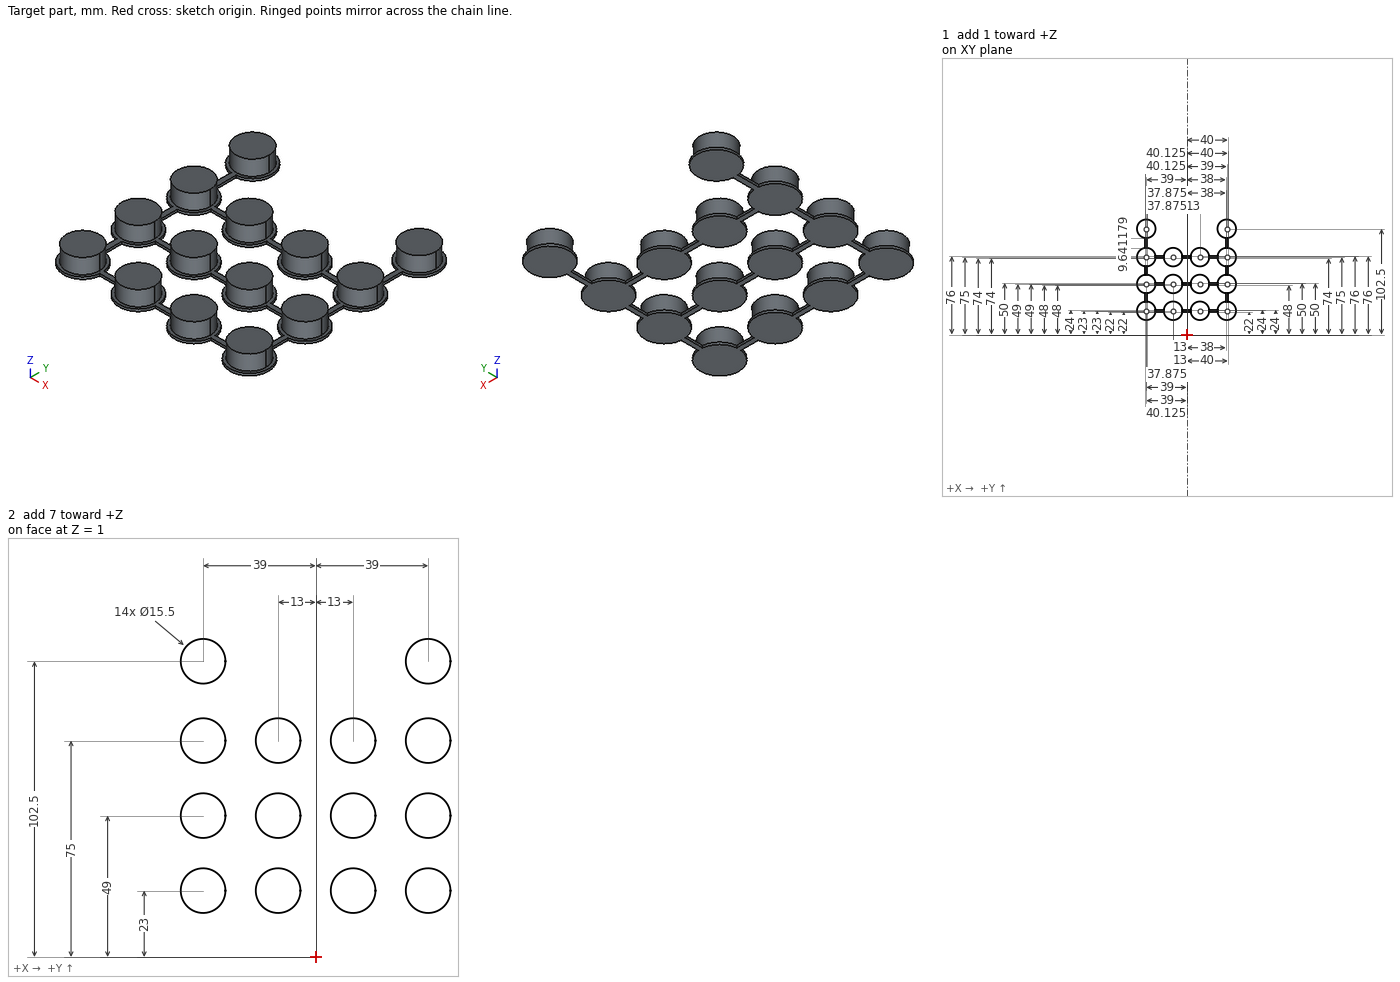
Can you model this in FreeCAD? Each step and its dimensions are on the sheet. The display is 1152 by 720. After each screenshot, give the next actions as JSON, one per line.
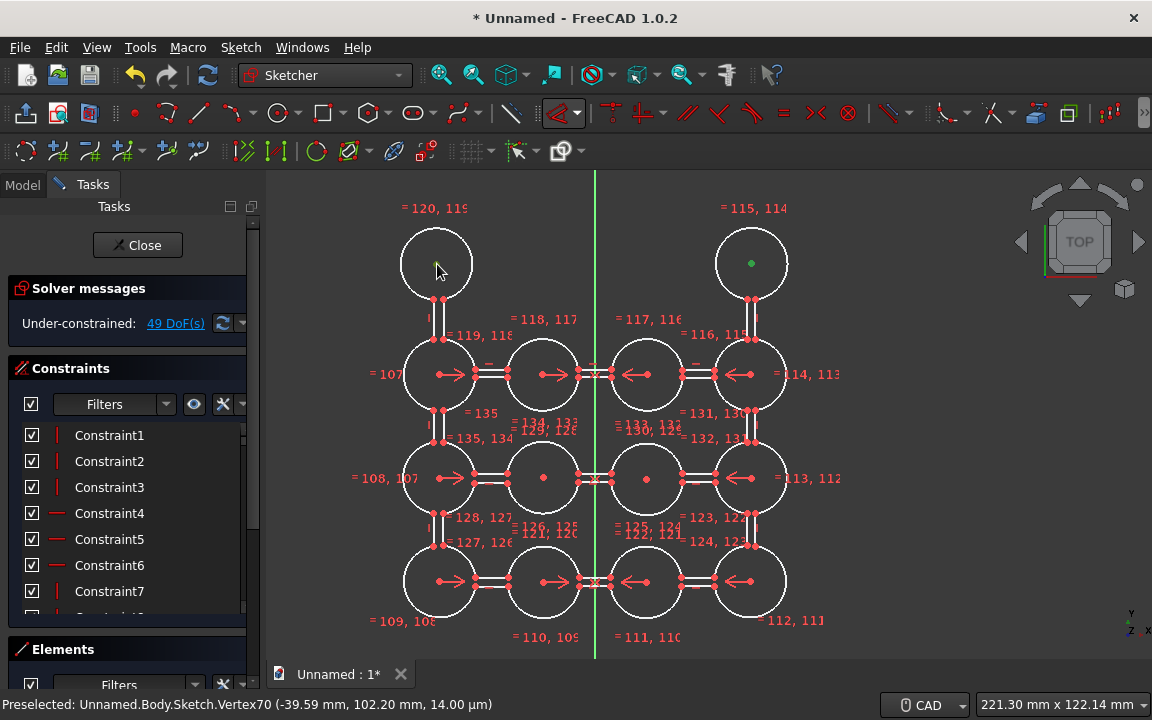
{"action": "left_click", "coordinate": [595, 538]}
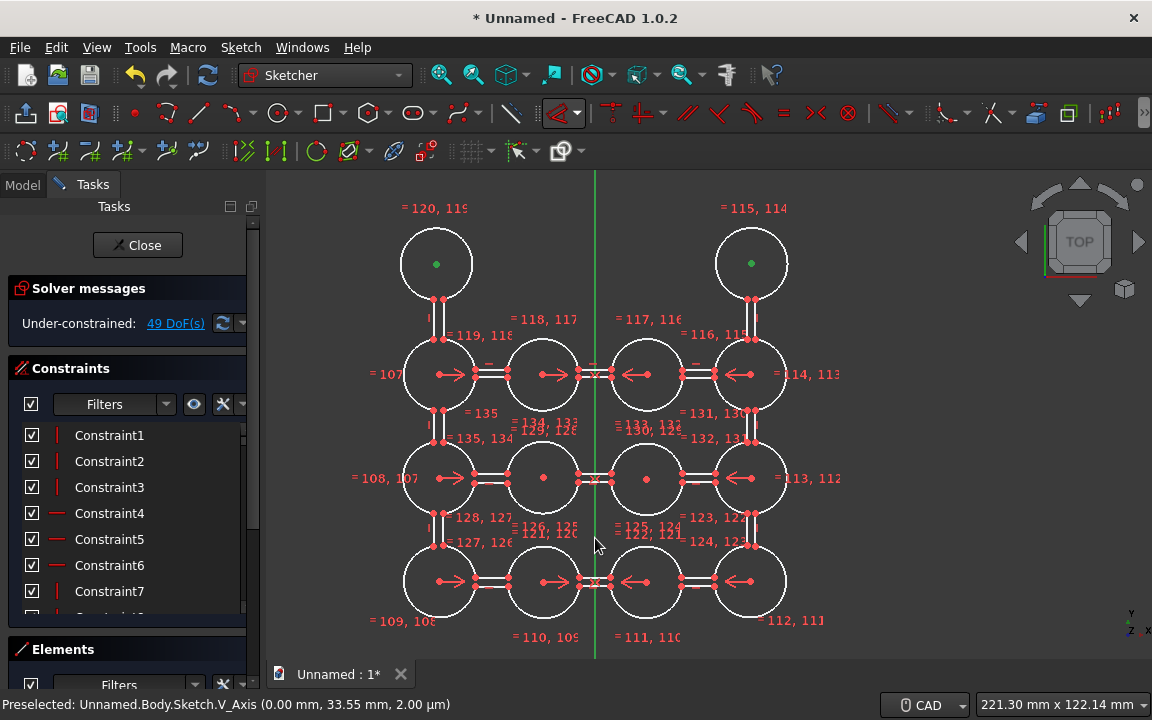
{"action": "left_click", "coordinate": [816, 114]}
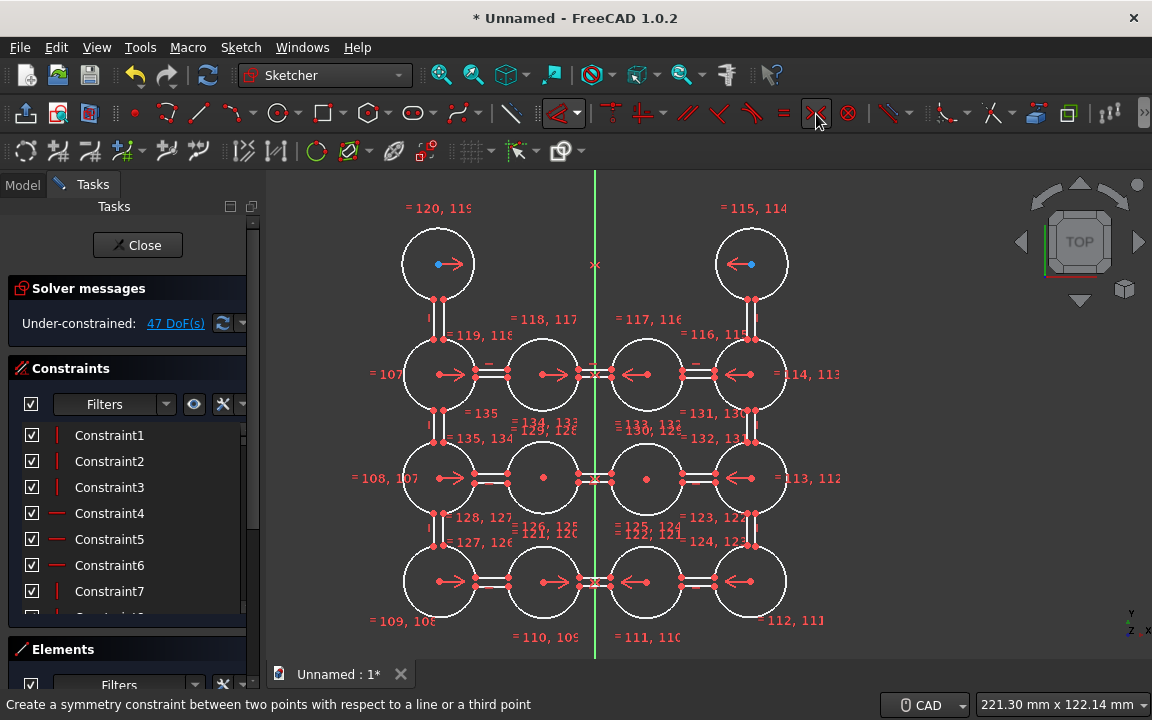
{"action": "left_click", "coordinate": [543, 478]}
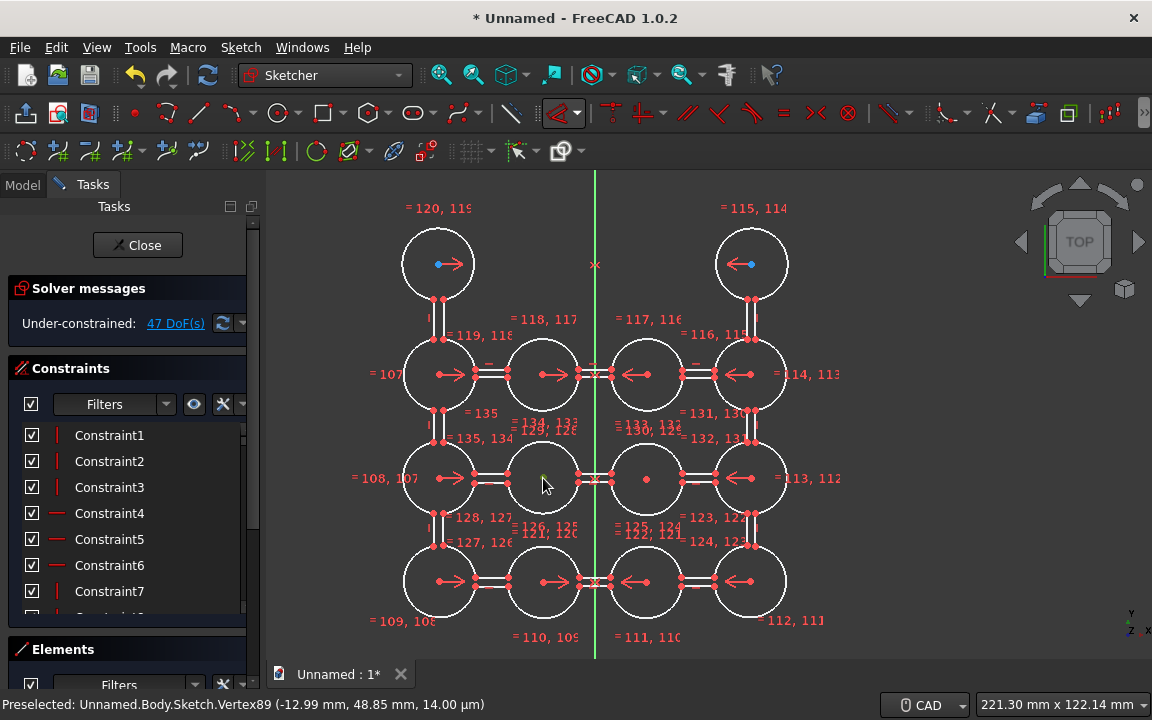
{"action": "left_click", "coordinate": [647, 479]}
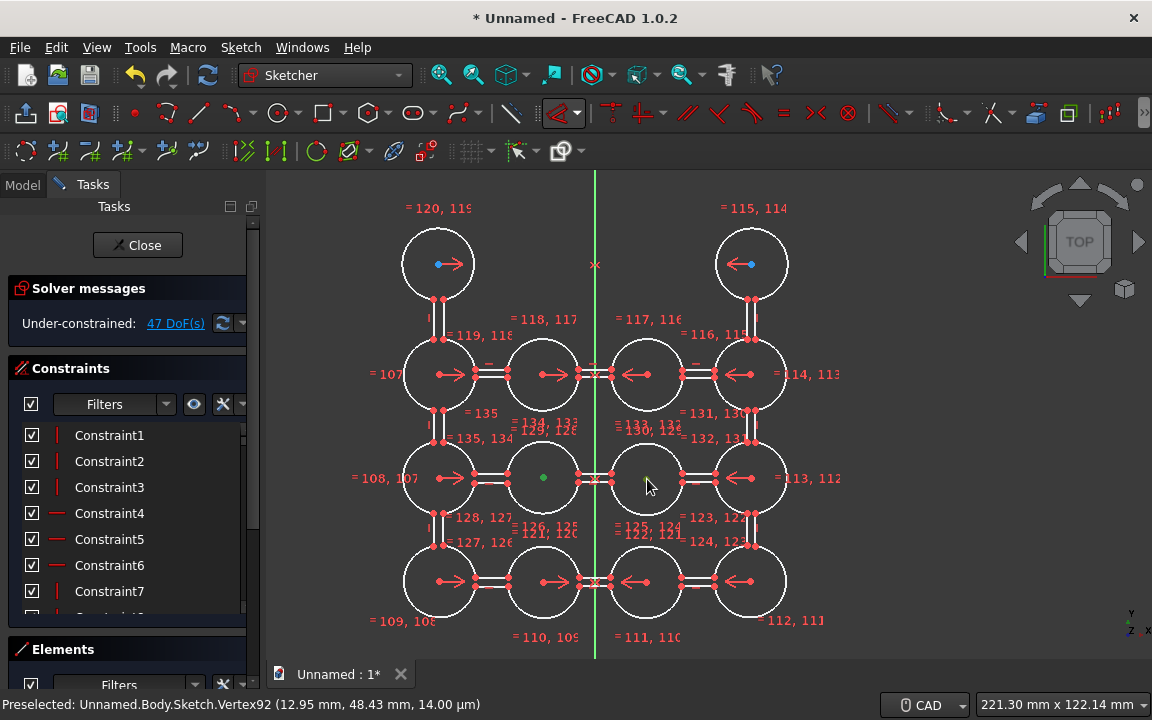
{"action": "left_click", "coordinate": [595, 538]}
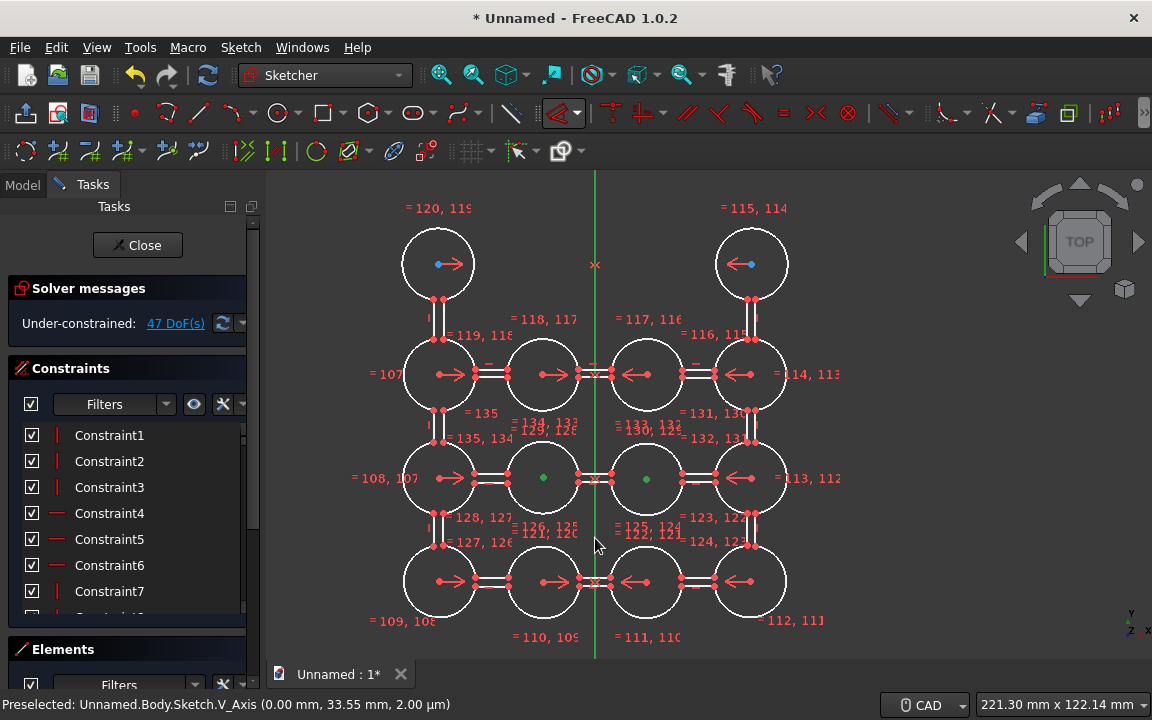
{"action": "left_click", "coordinate": [816, 114]}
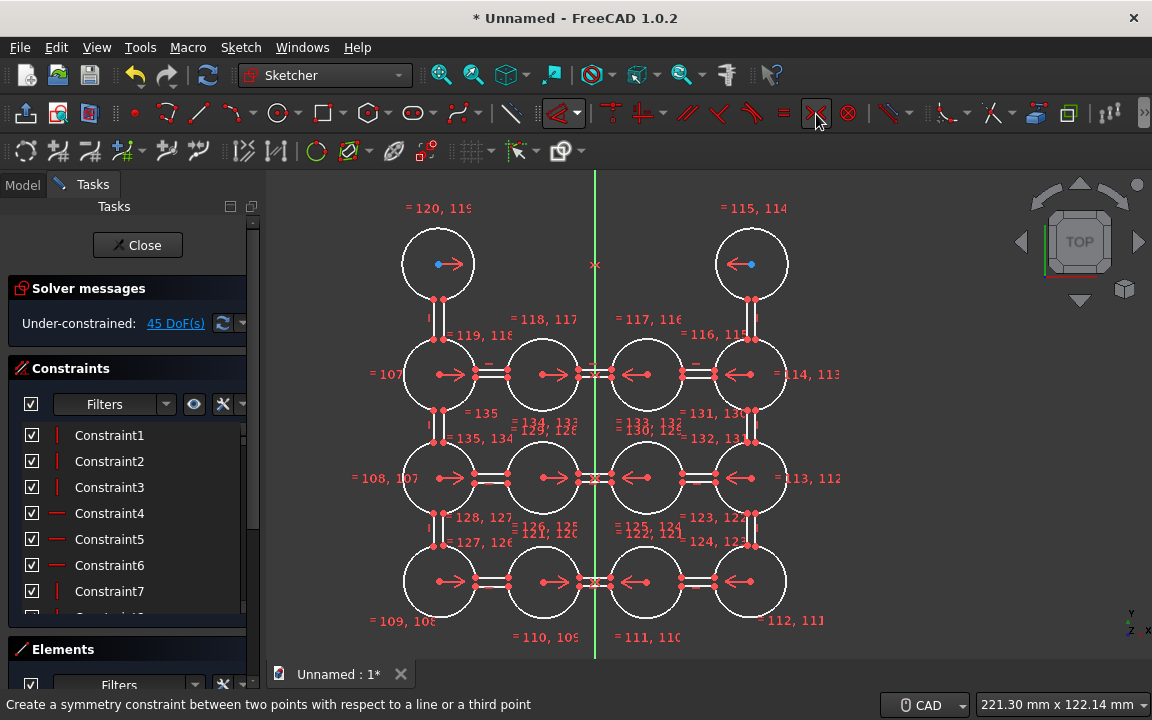
{"action": "scroll", "coordinate": [475, 587], "scroll_direction": "up", "scroll_amount": 2}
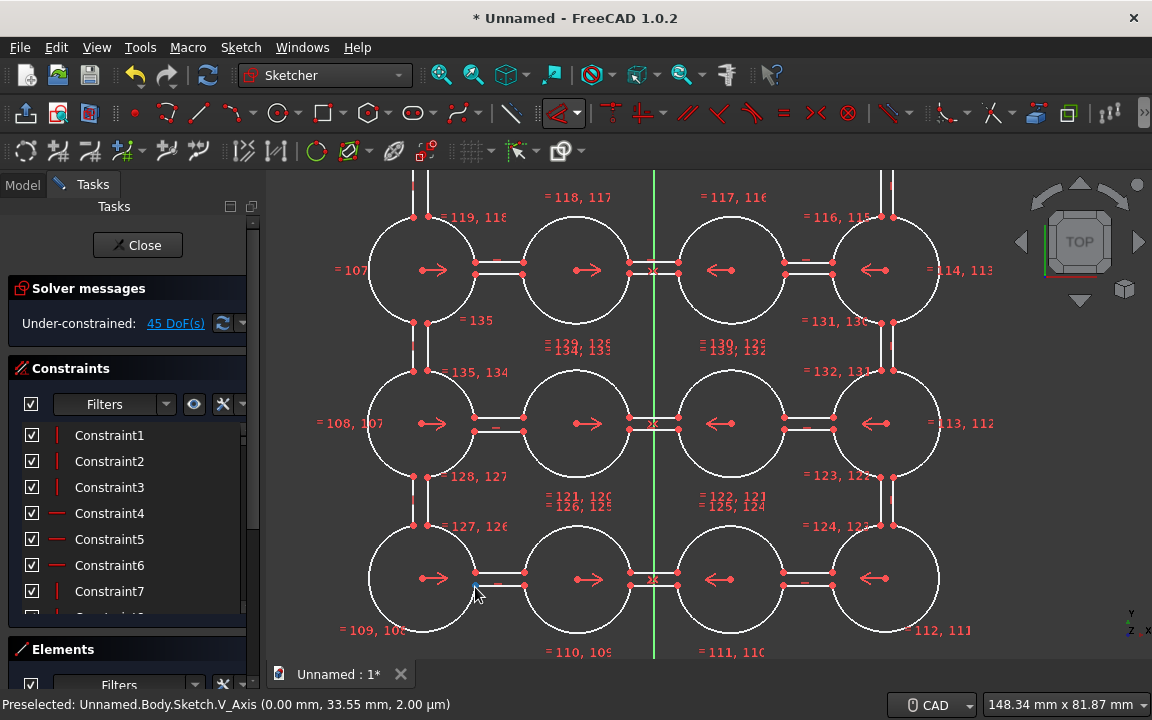
{"action": "left_click", "coordinate": [475, 586]}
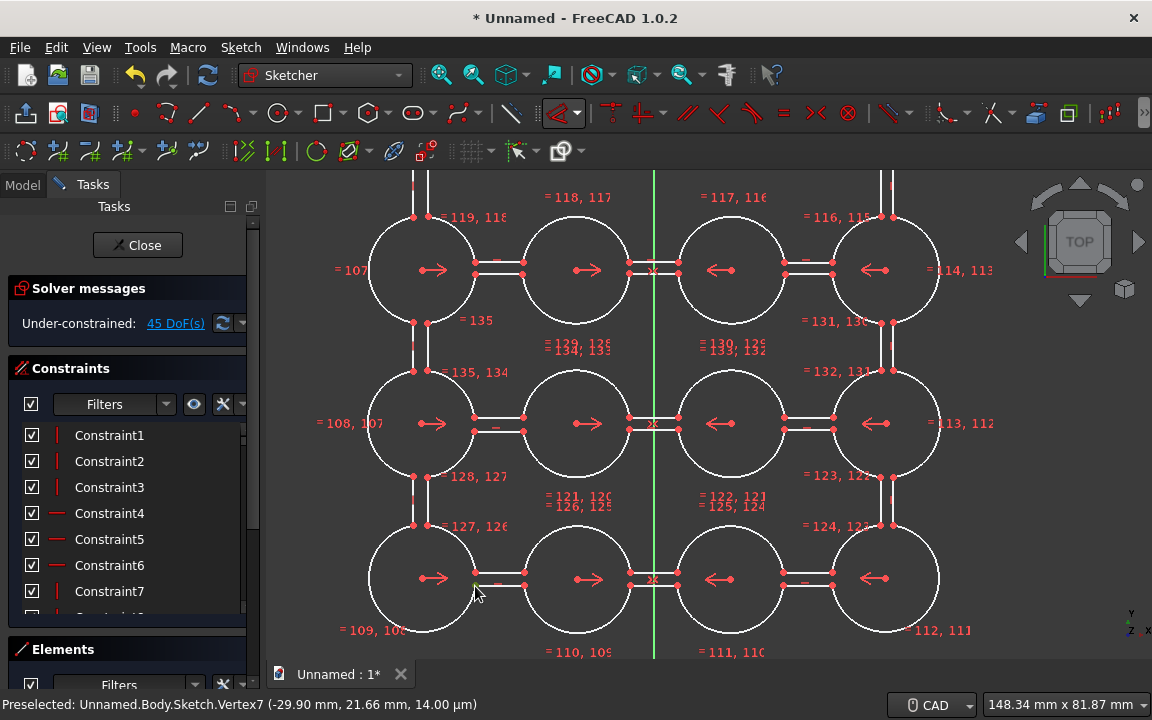
{"action": "left_click", "coordinate": [580, 114]}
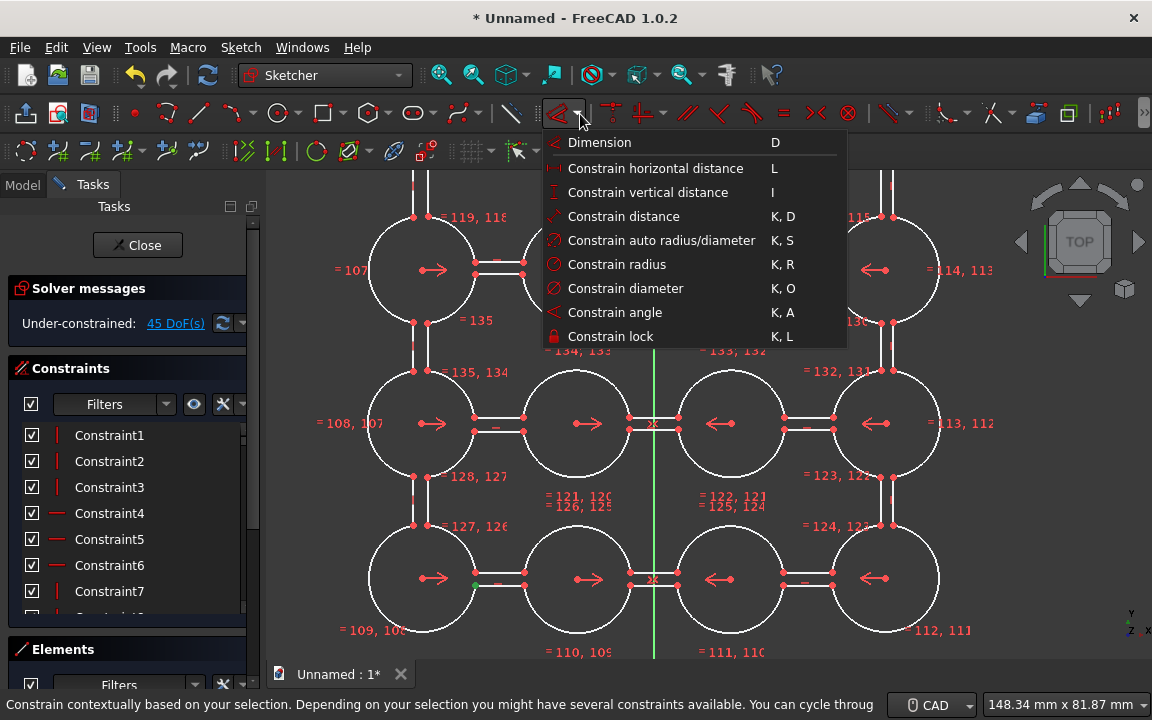
{"action": "left_click", "coordinate": [695, 192]}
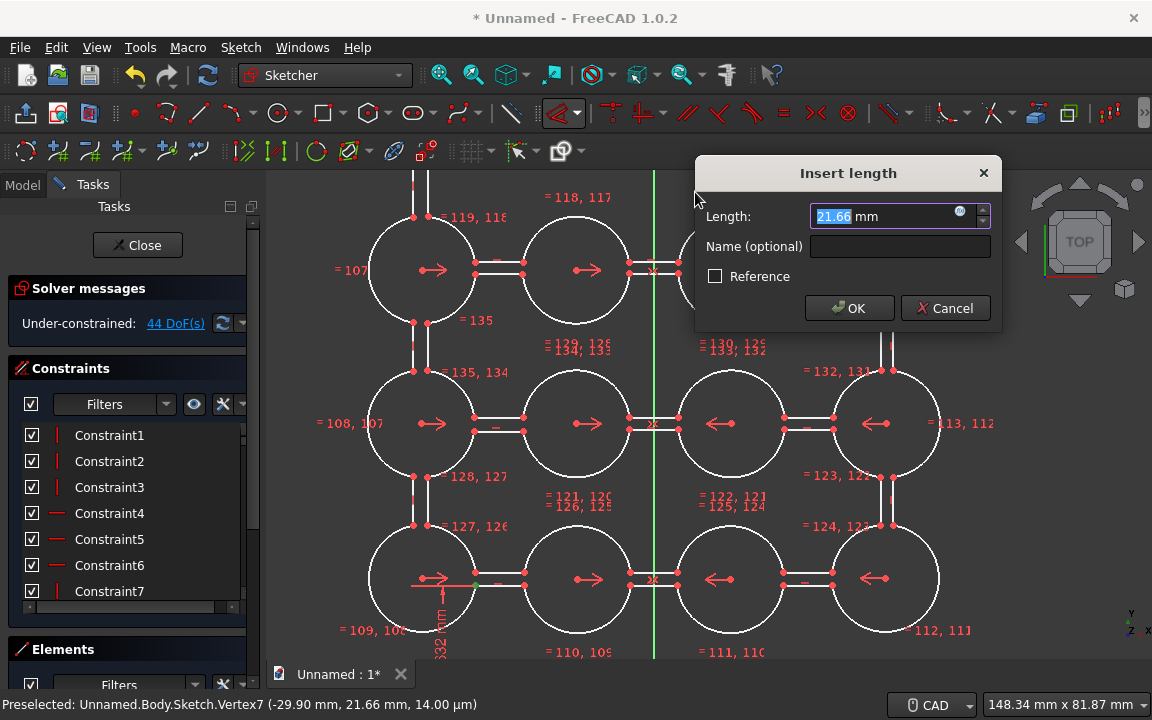
{"action": "type", "text": "22"}
{"action": "key", "text": "Return"}